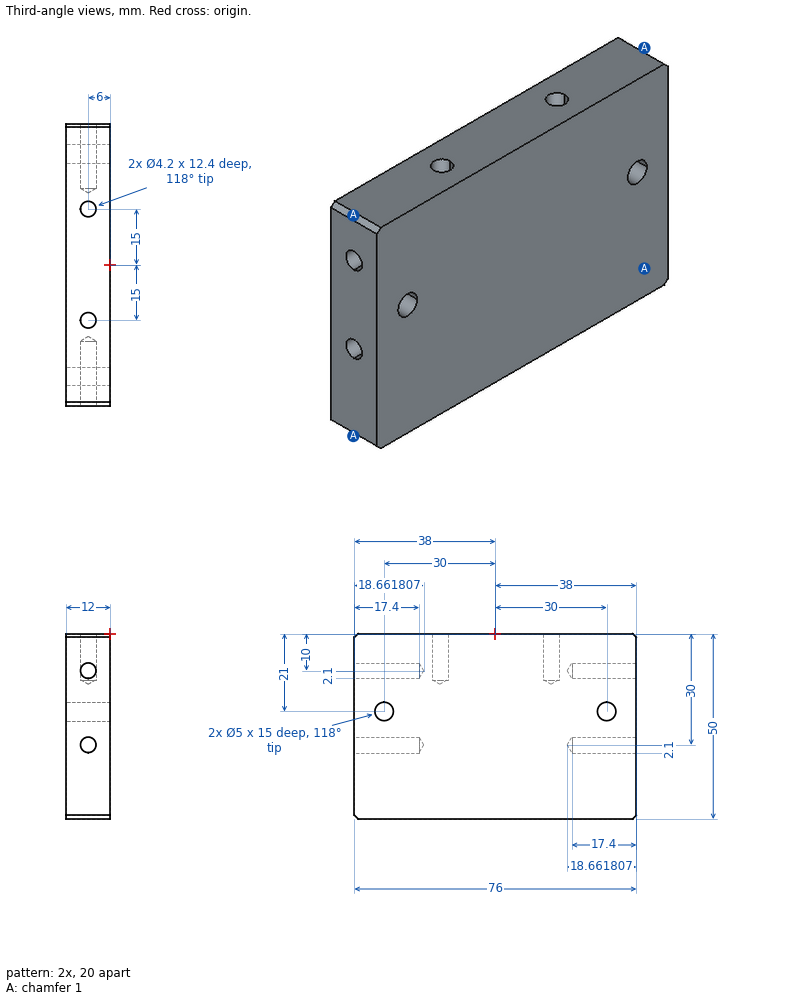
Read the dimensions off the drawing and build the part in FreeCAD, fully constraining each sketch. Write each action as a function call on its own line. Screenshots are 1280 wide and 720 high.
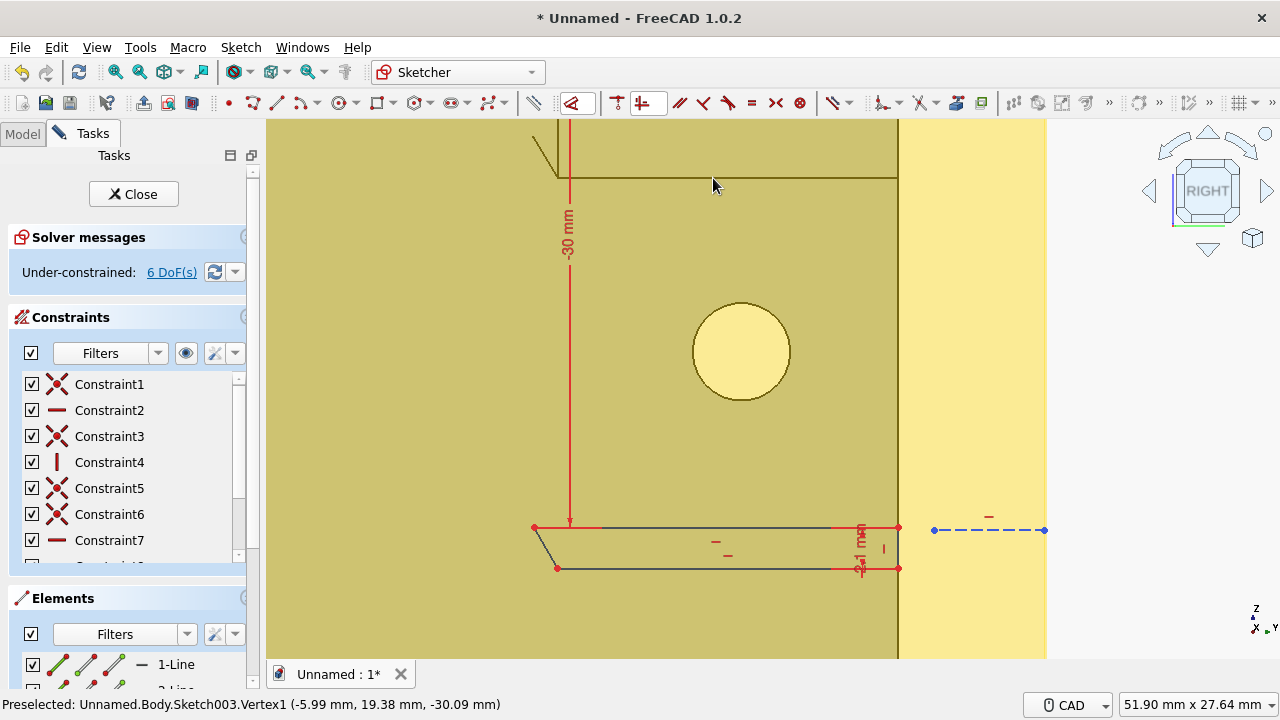
click(898, 569)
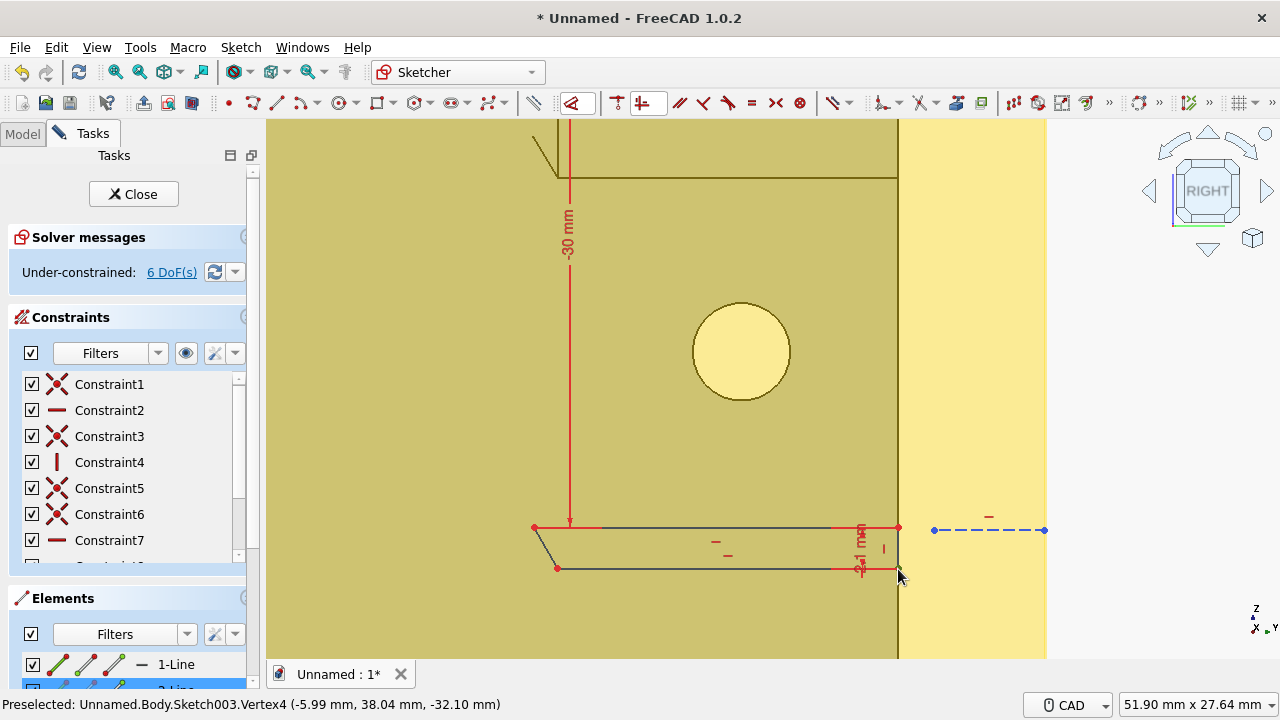
key(l)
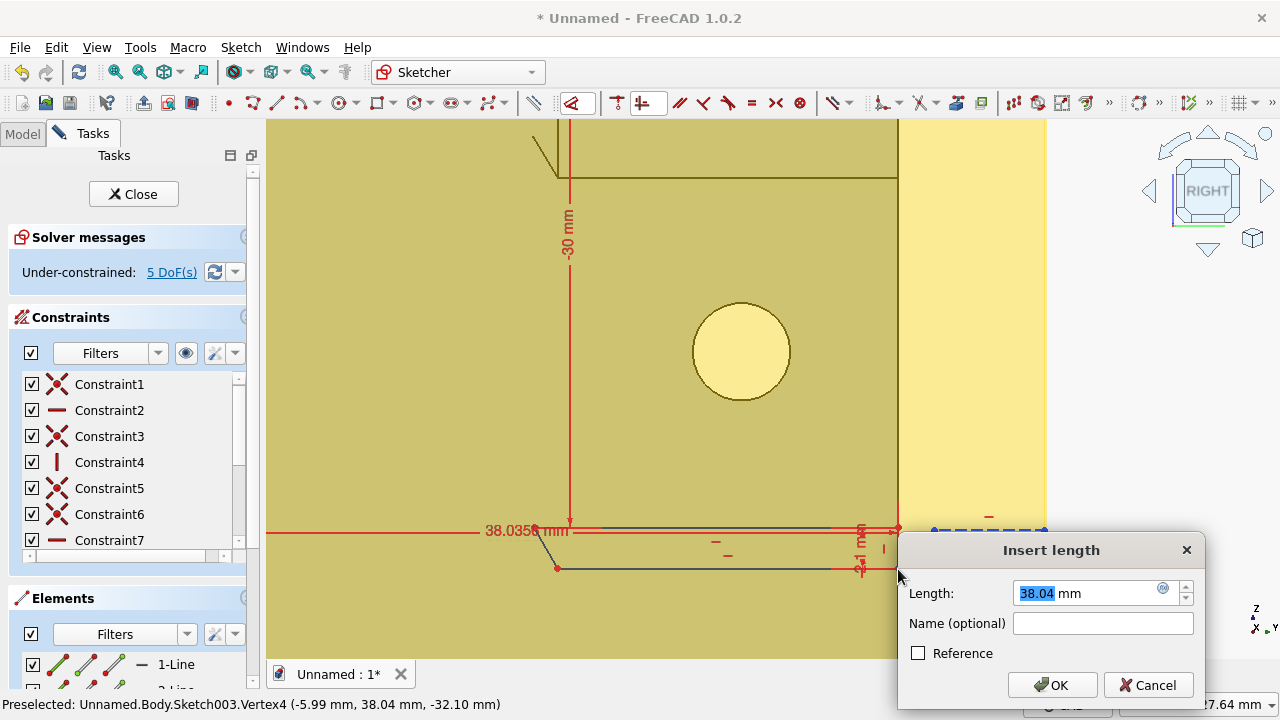
text(38)
key(Return)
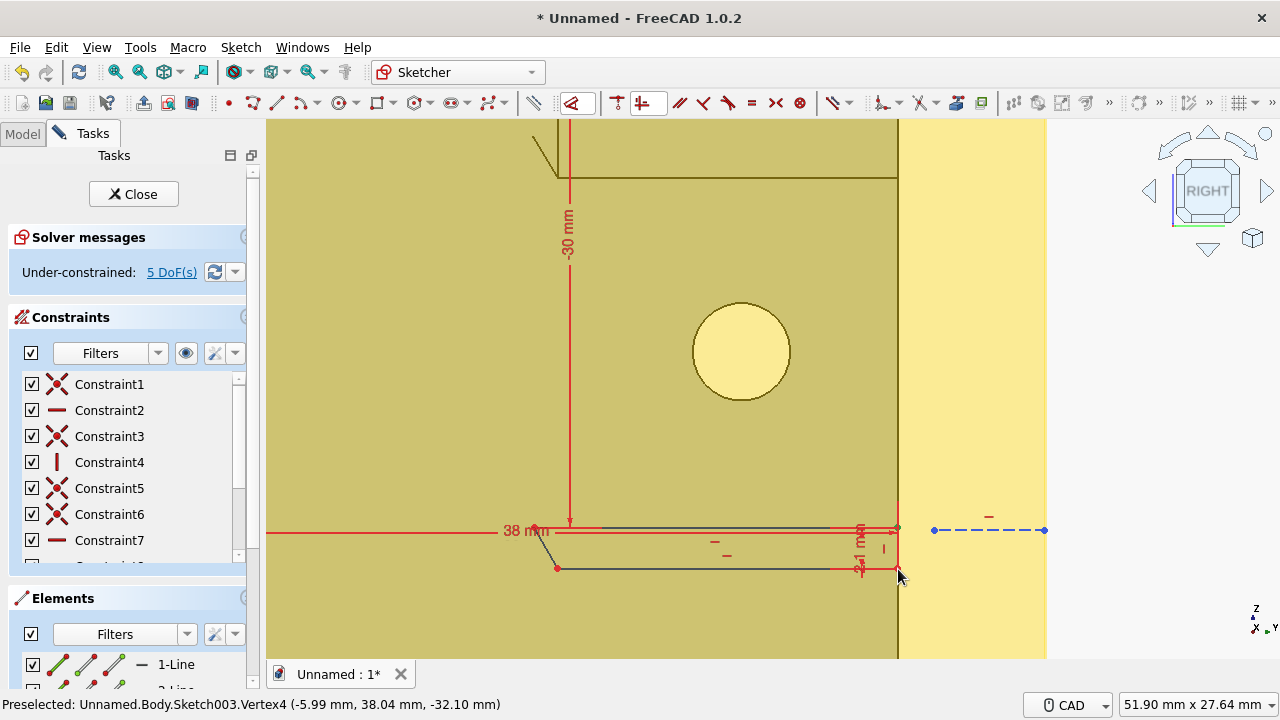
click(935, 530)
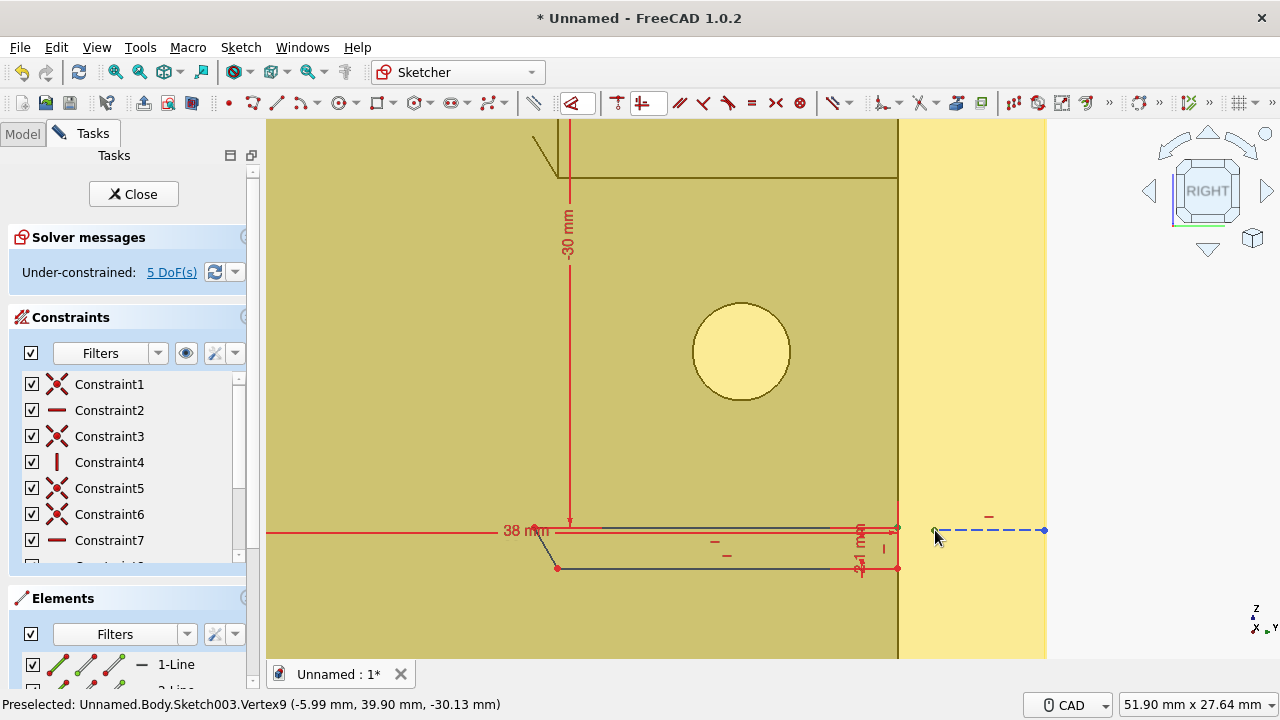
click(590, 104)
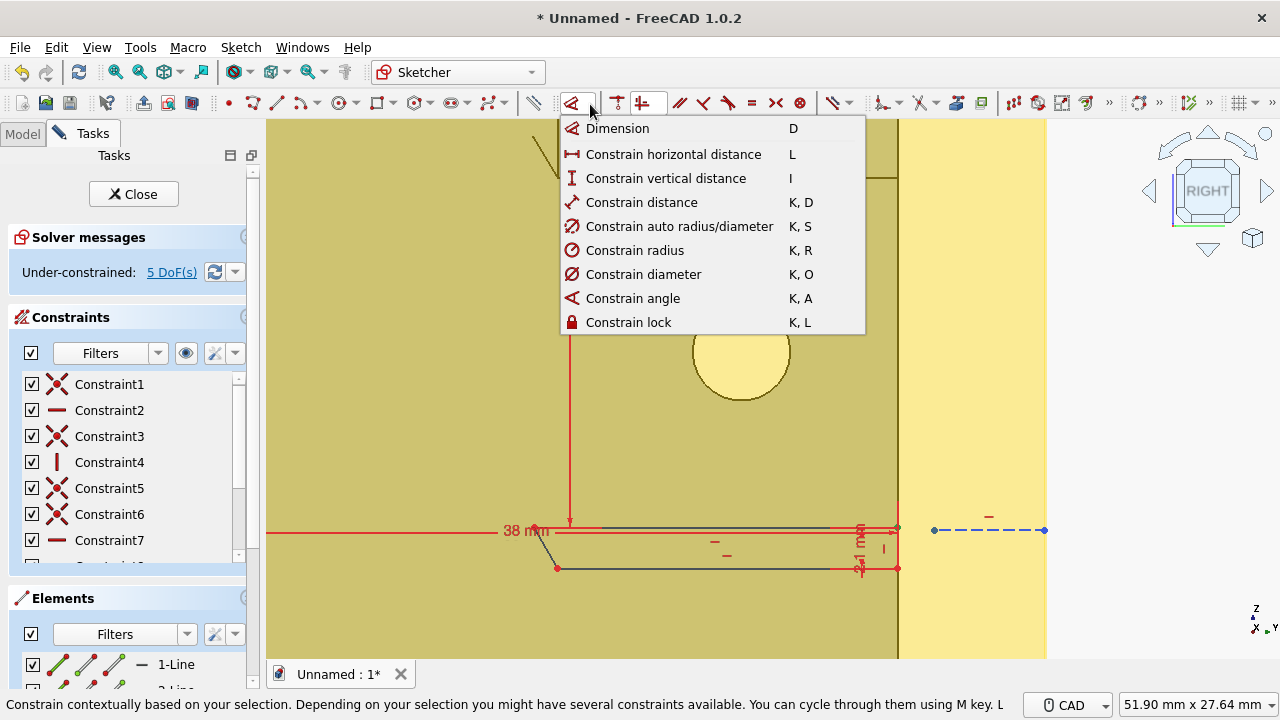
click(713, 178)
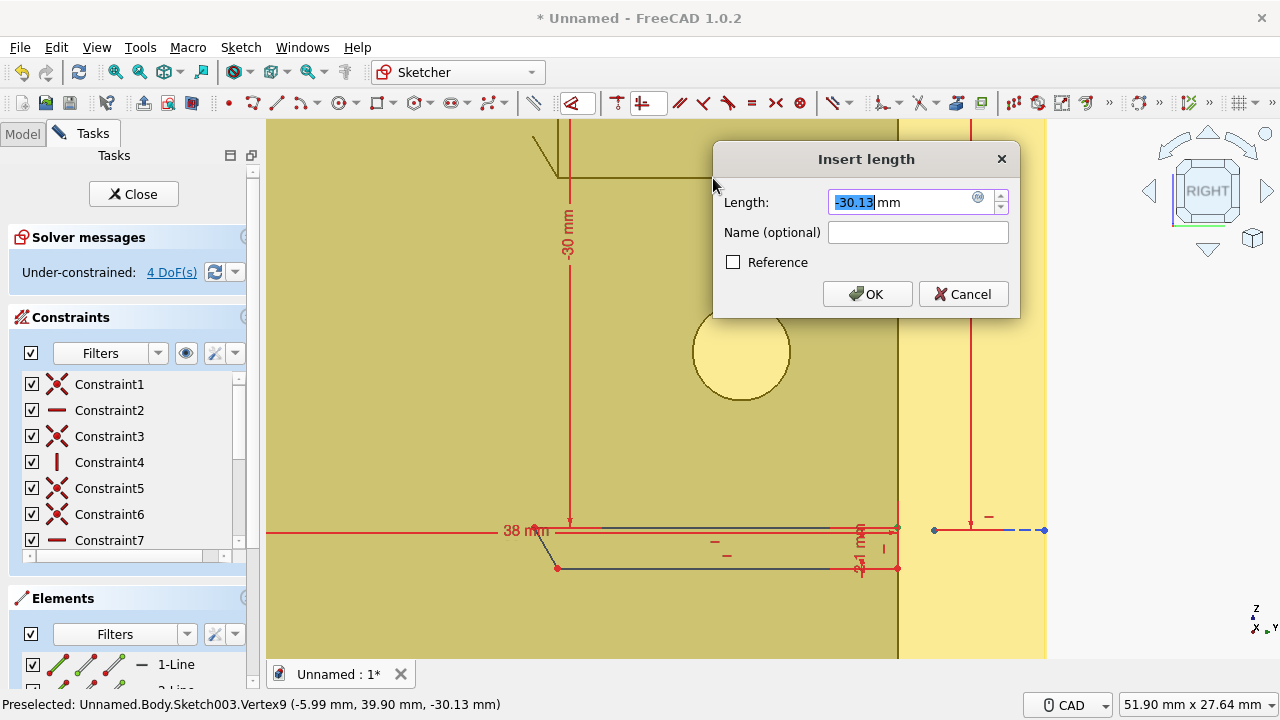
text(-30)
key(Return)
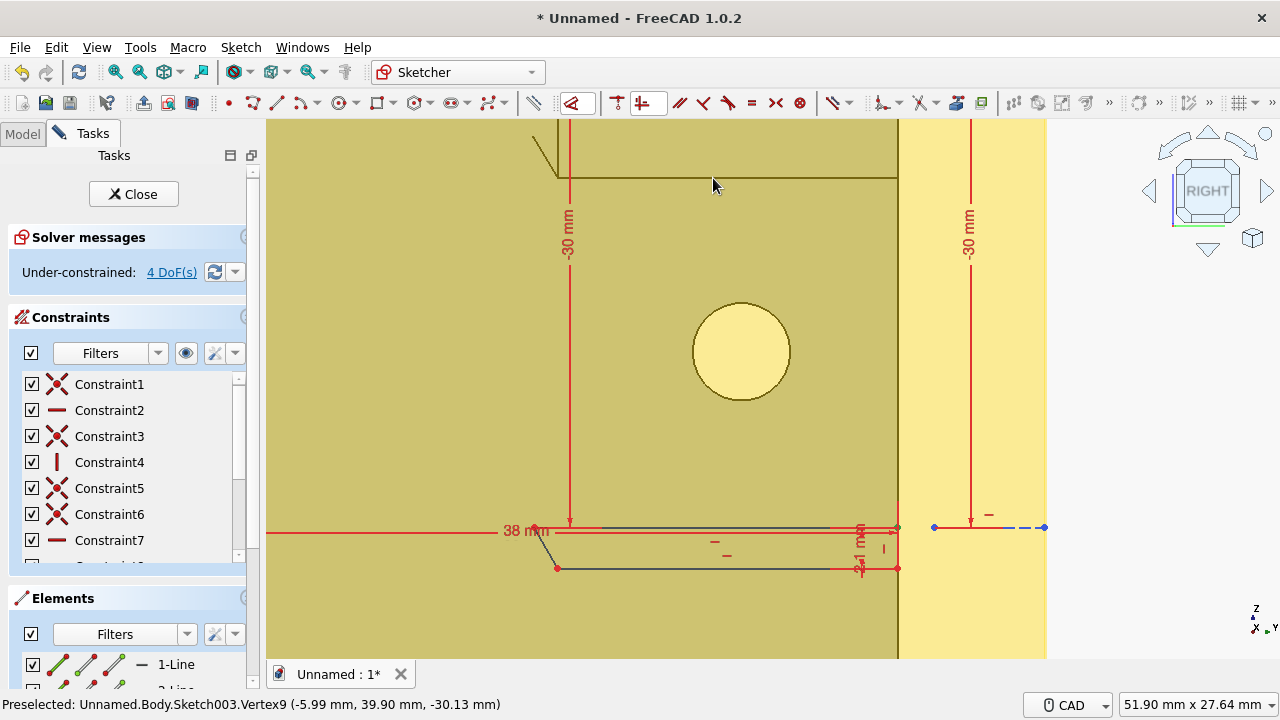
click(660, 569)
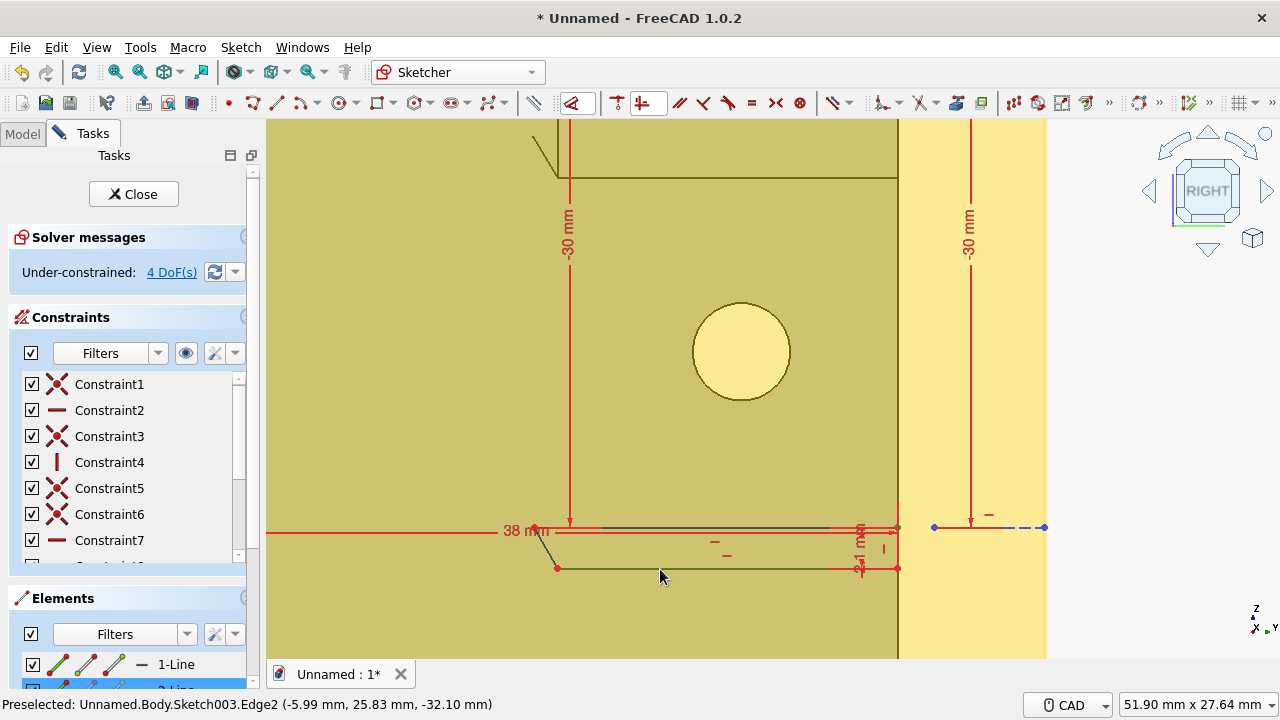
click(590, 104)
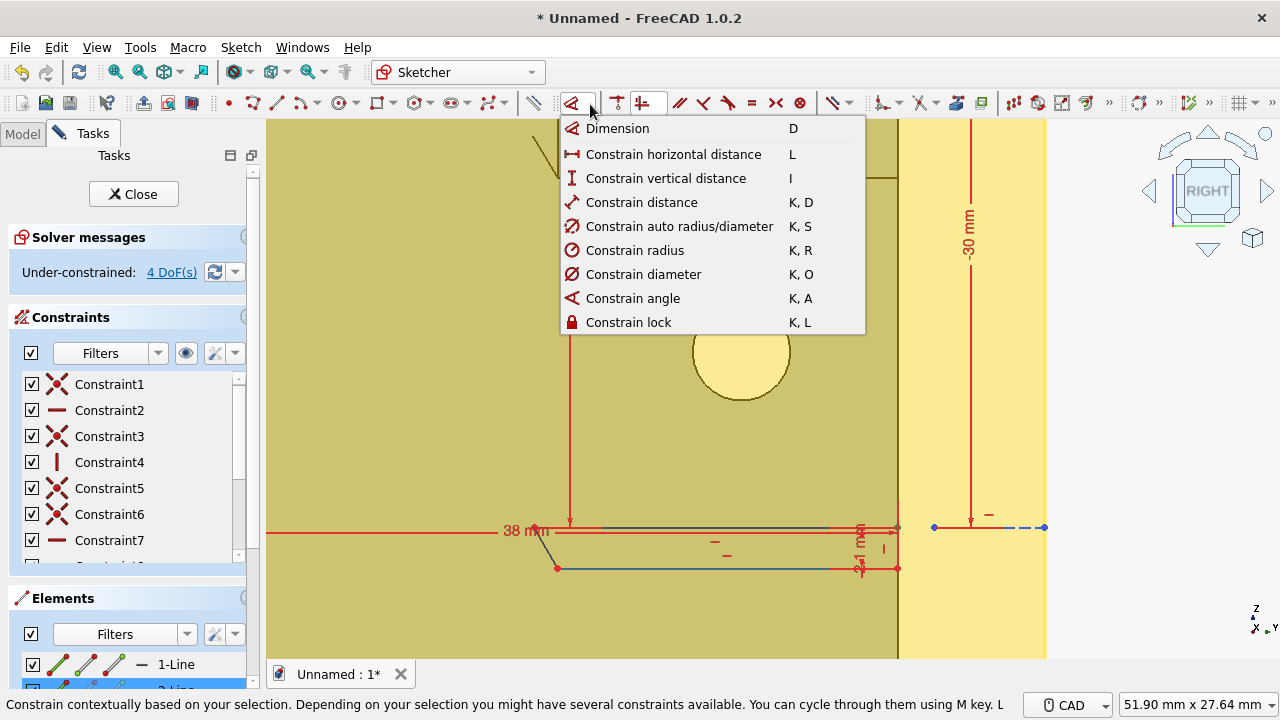
click(713, 154)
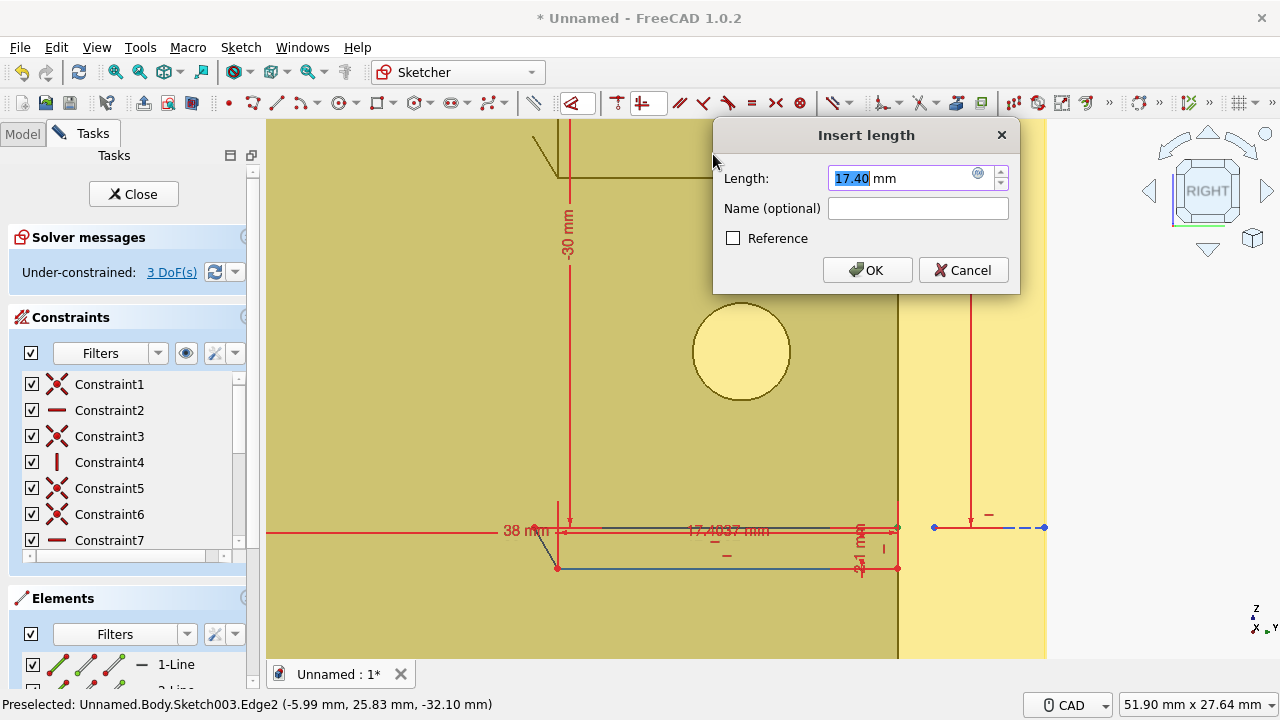
text(17.4)
key(Return)